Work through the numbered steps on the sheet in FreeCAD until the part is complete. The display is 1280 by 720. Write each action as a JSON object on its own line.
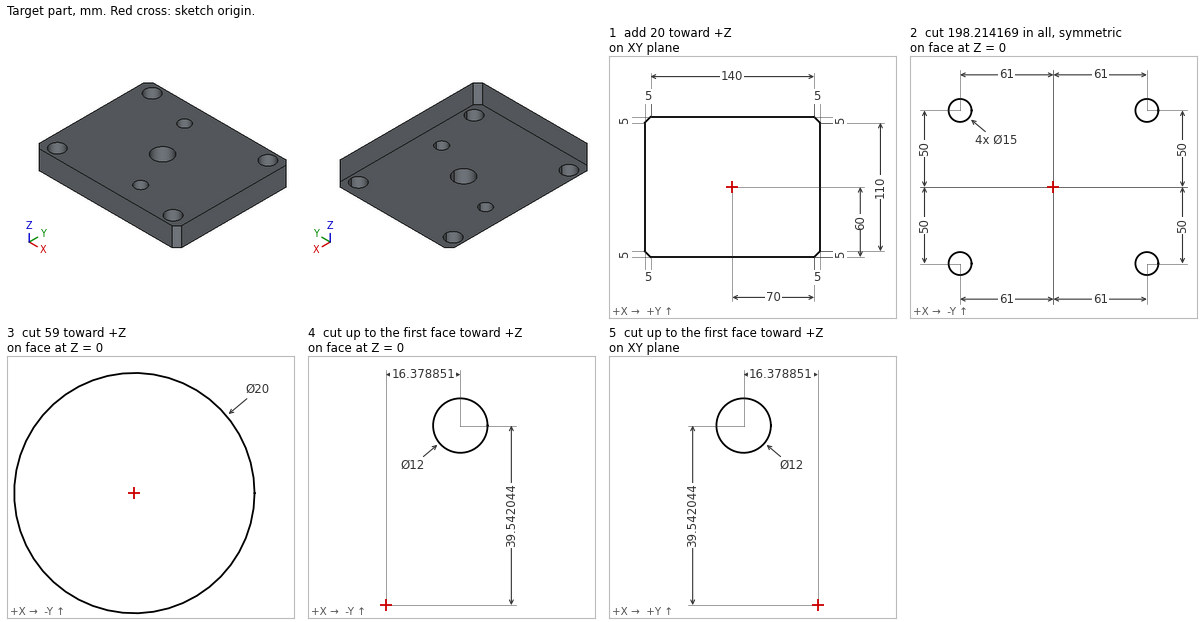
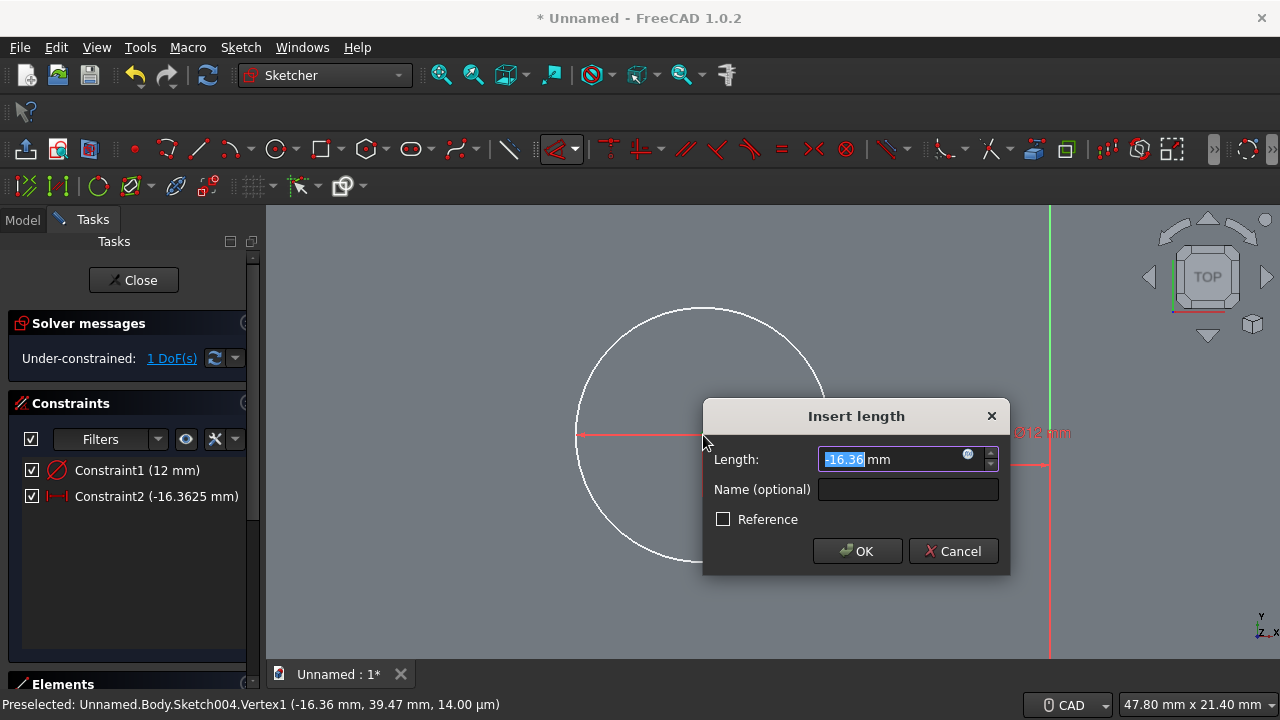
{"action": "type", "text": "-16.378851"}
{"action": "key", "text": "Return"}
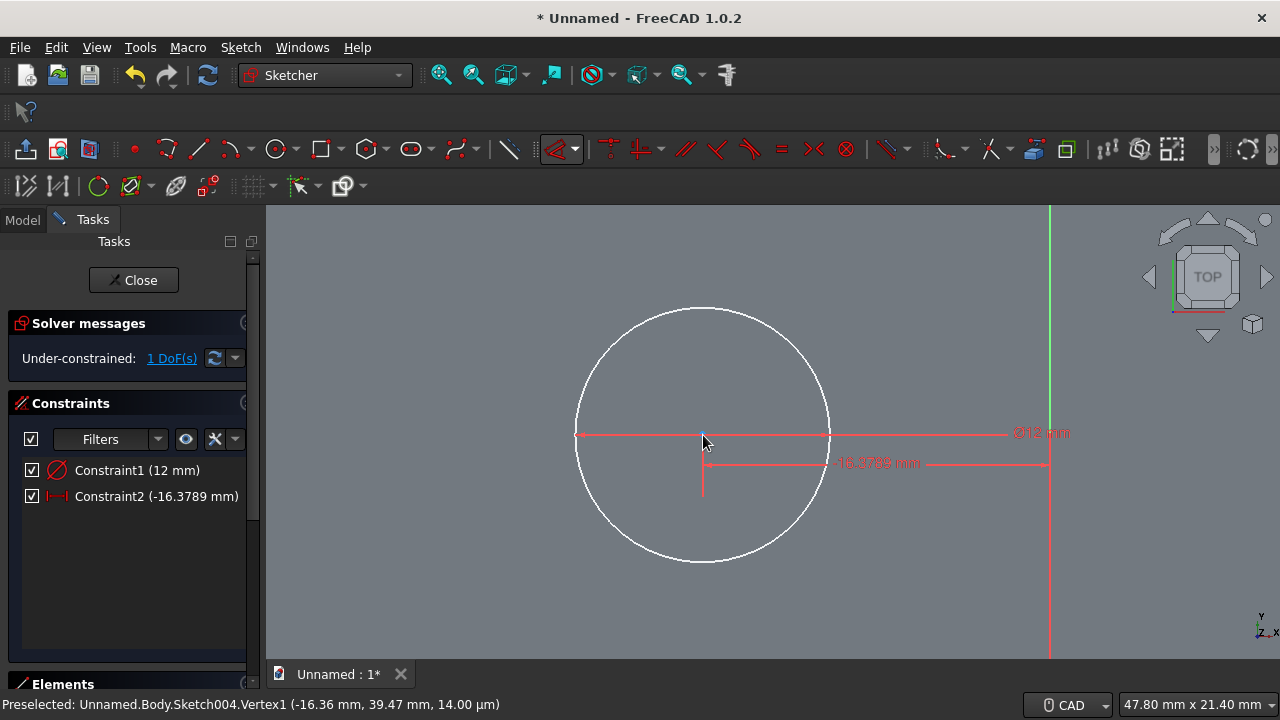
{"action": "left_click", "coordinate": [703, 435]}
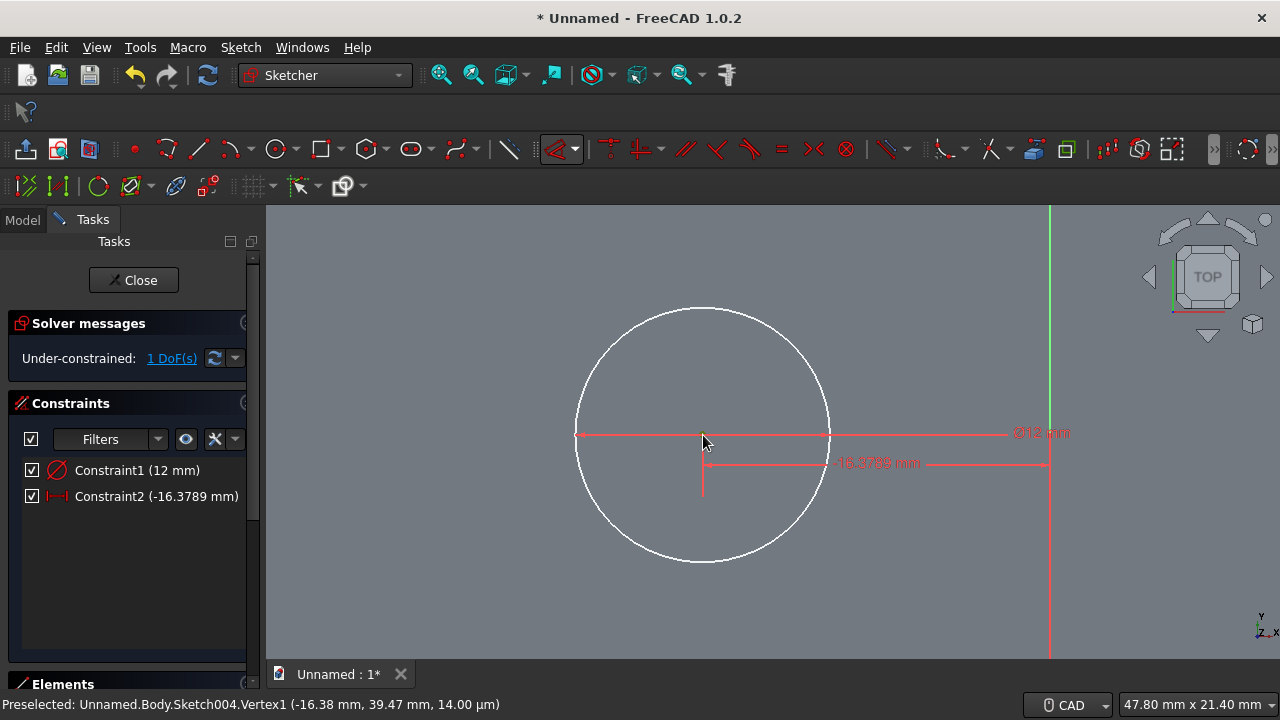
{"action": "left_click", "coordinate": [578, 150]}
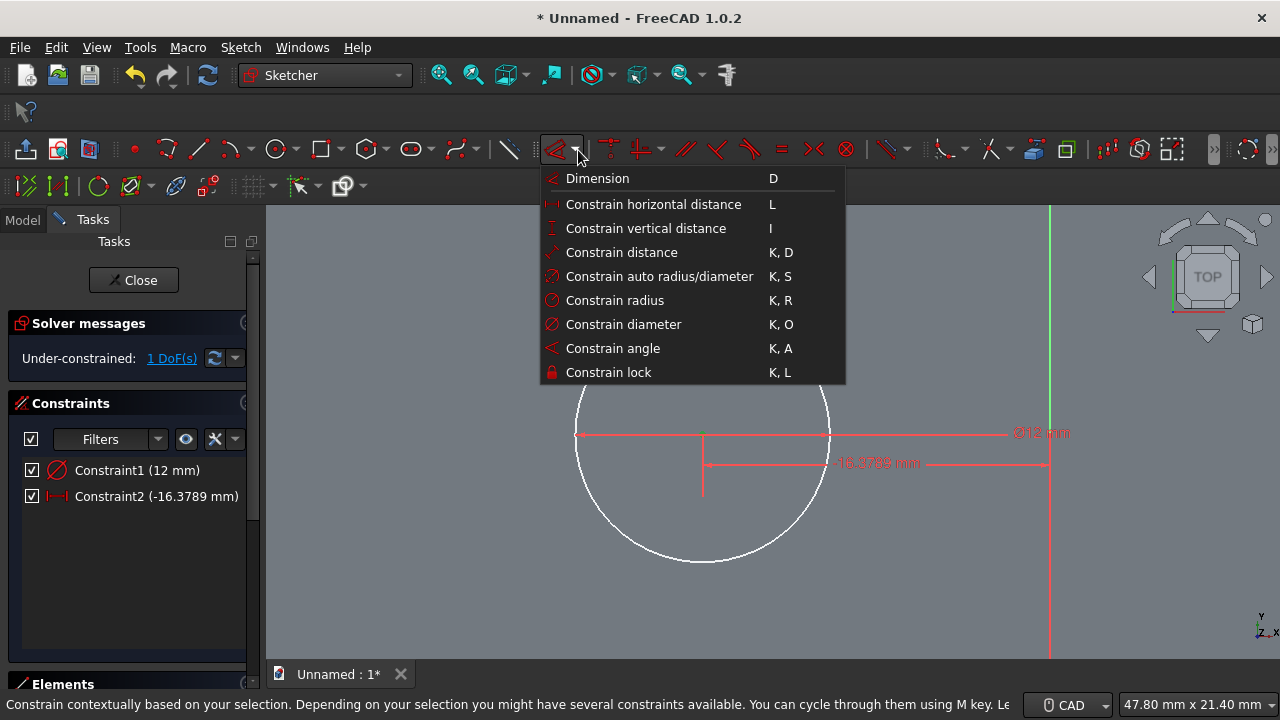
{"action": "left_click", "coordinate": [693, 228]}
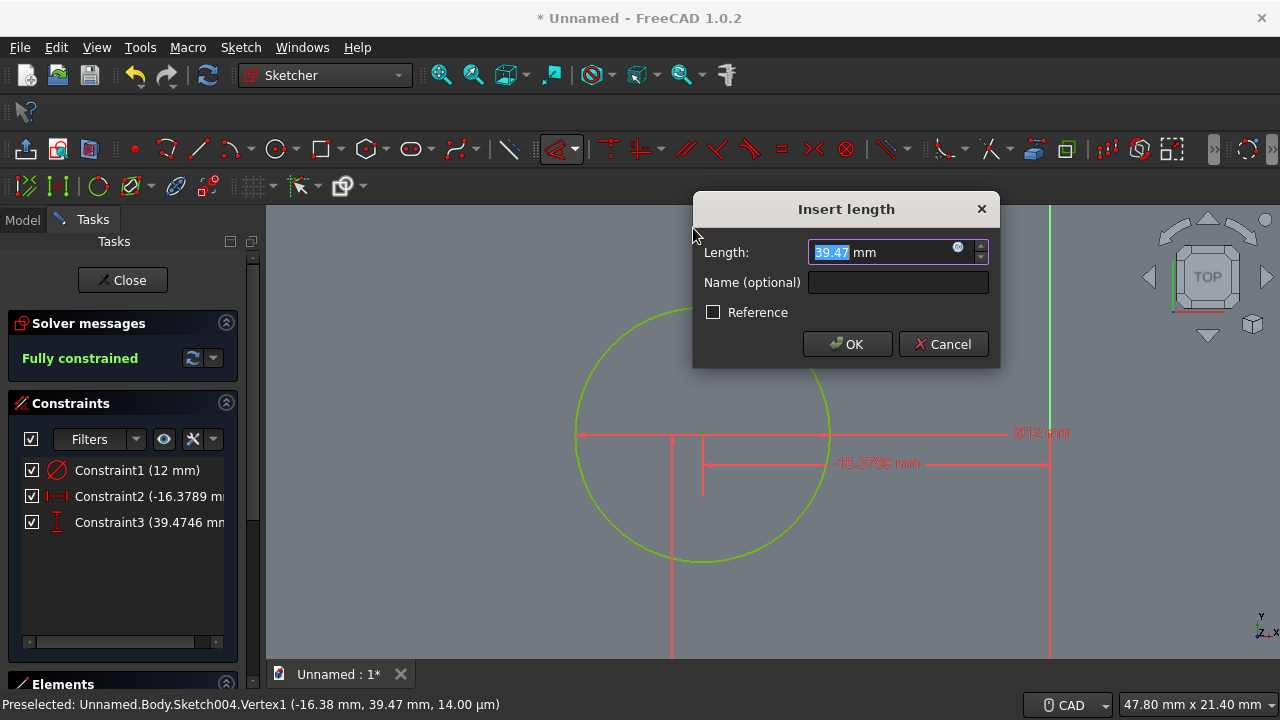
{"action": "type", "text": "39.542044"}
{"action": "key", "text": "Return"}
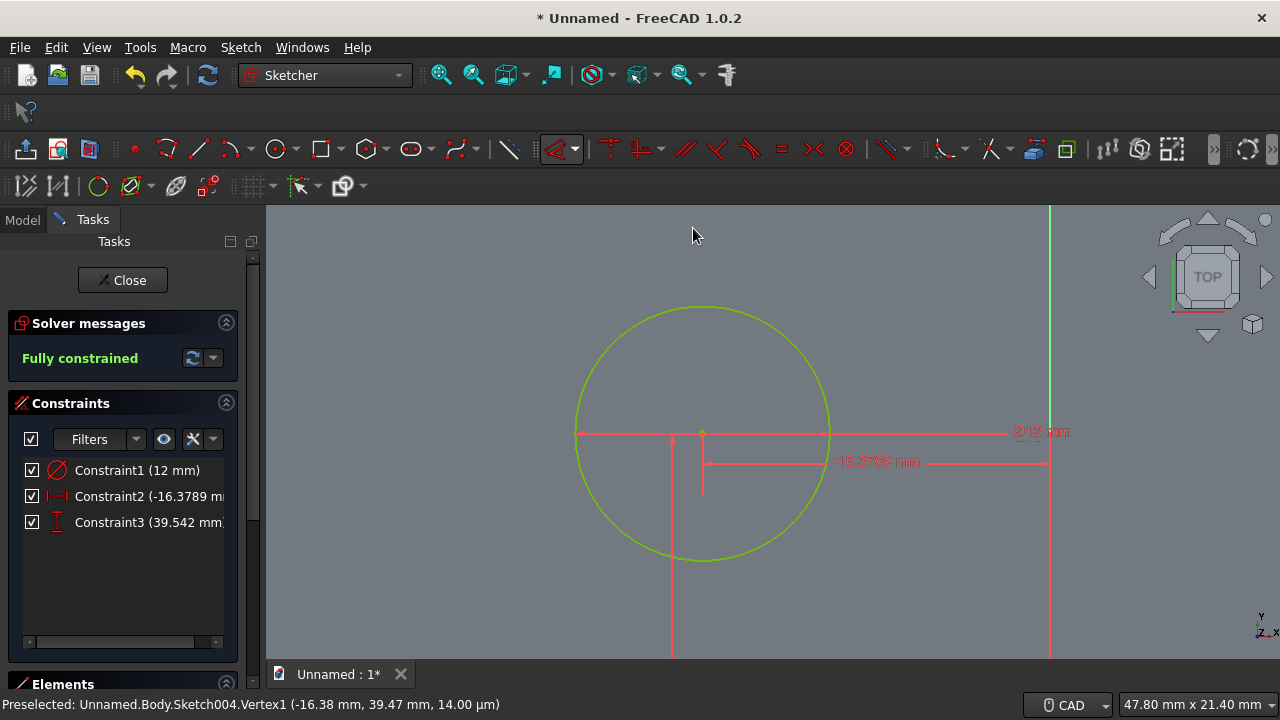
{"action": "left_click", "coordinate": [123, 280]}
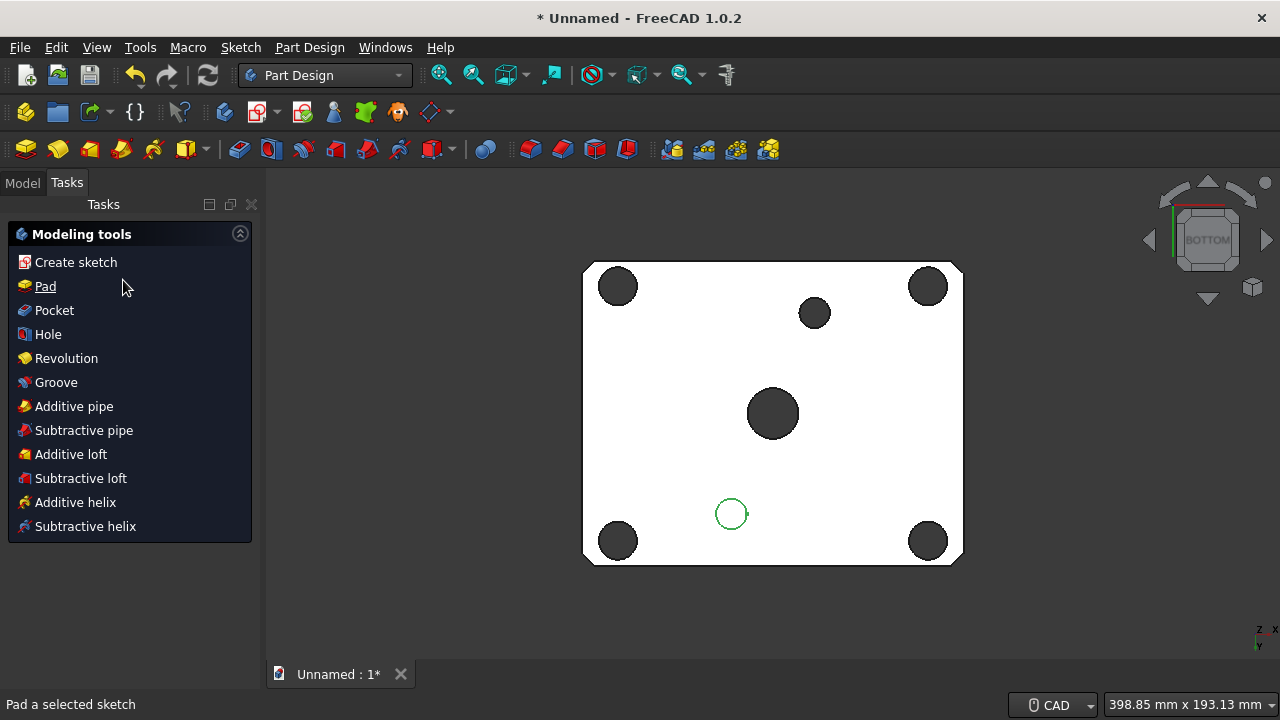
{"action": "left_click", "coordinate": [240, 150]}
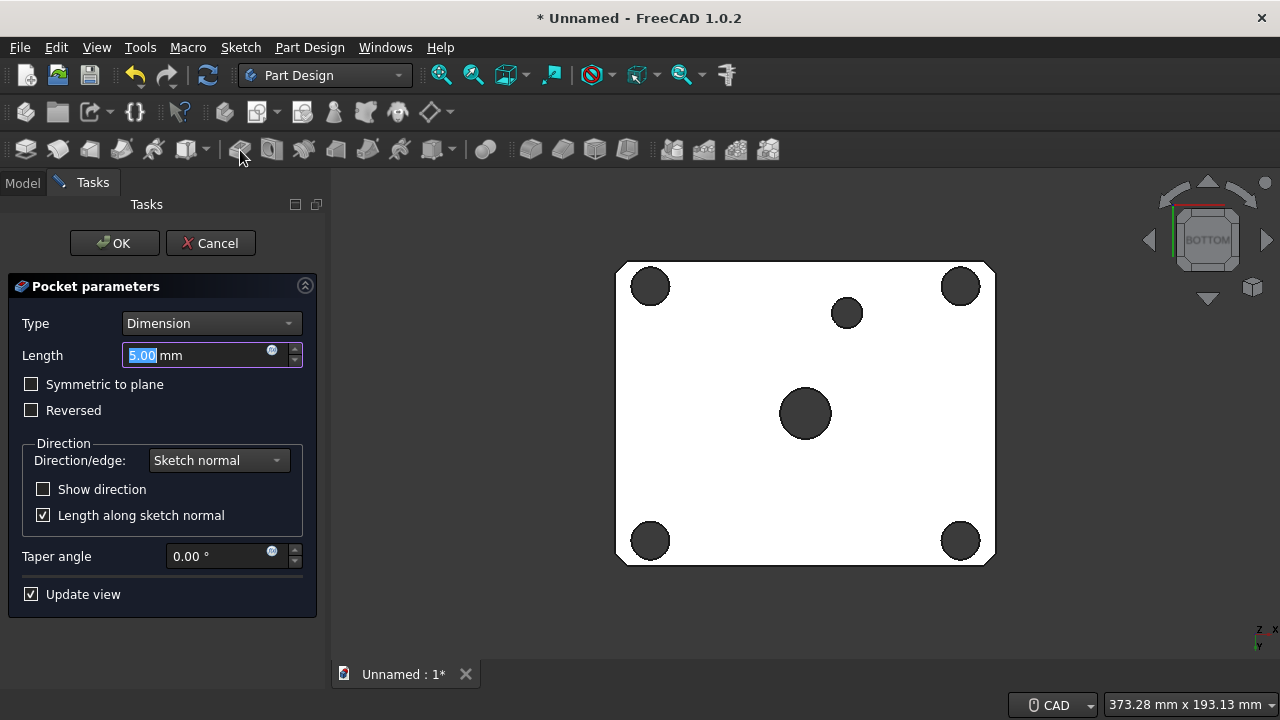
{"action": "left_click", "coordinate": [212, 324]}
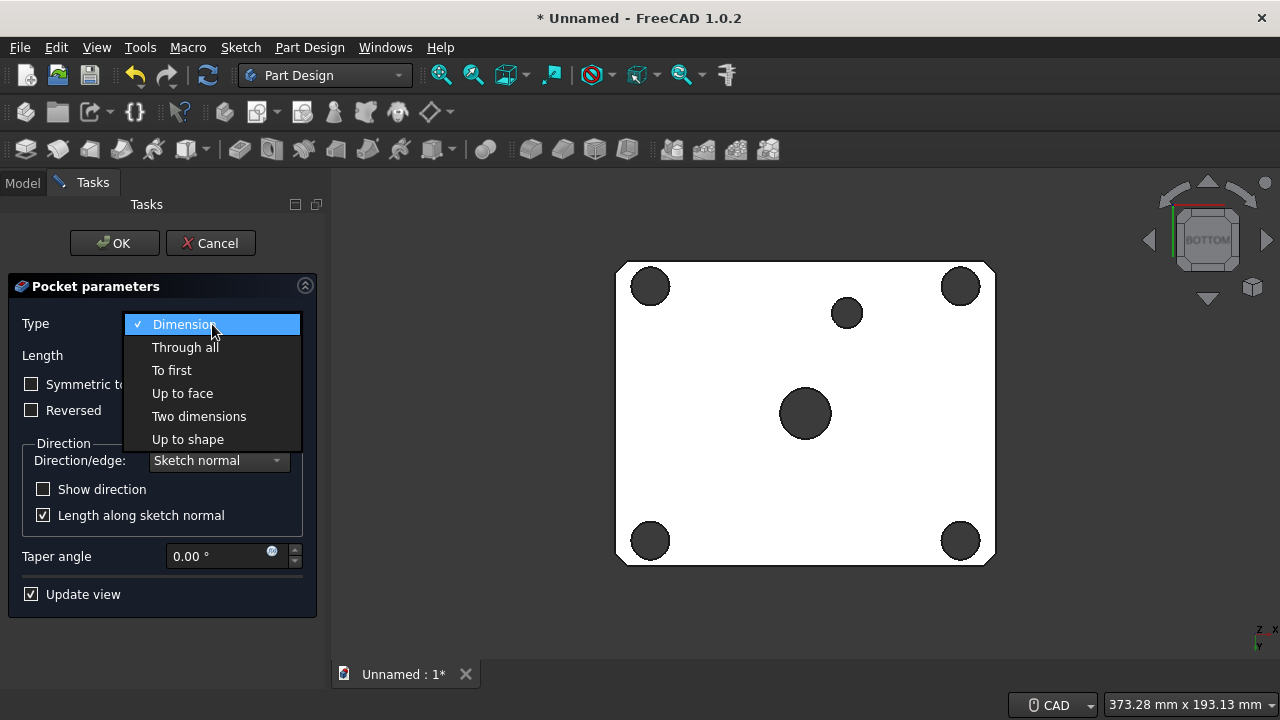
{"action": "left_click", "coordinate": [212, 370]}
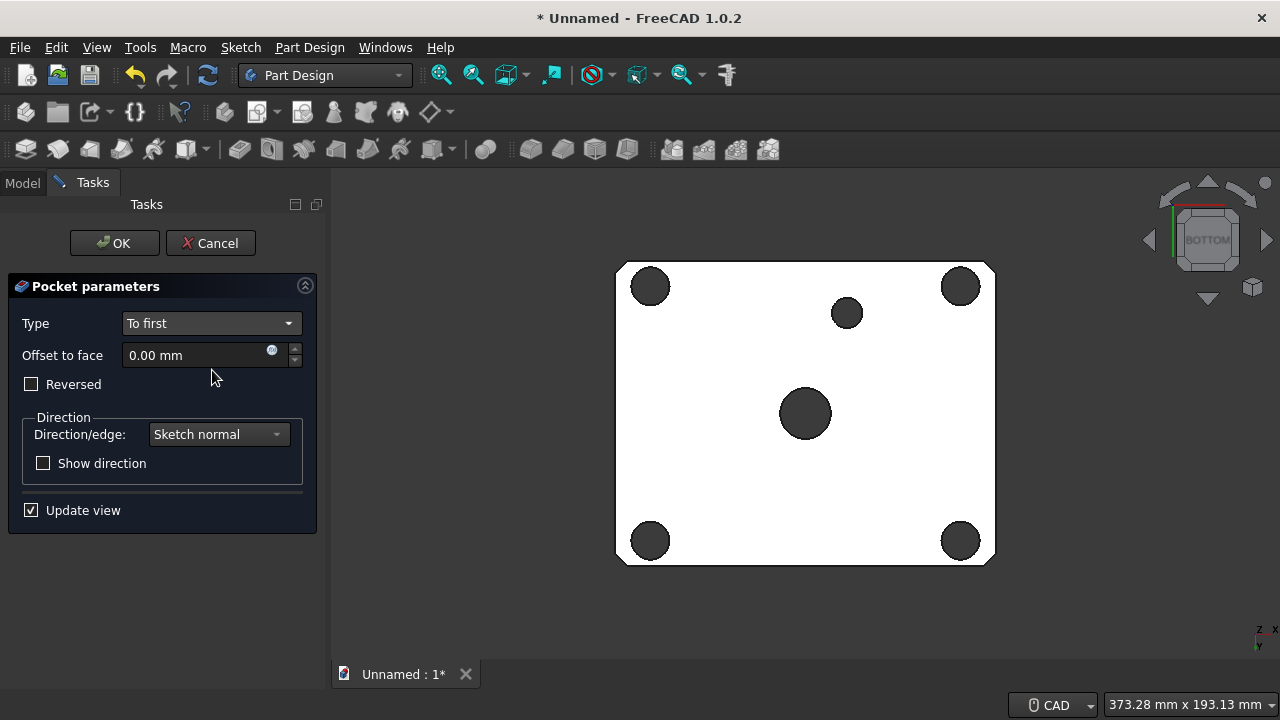
{"action": "left_click", "coordinate": [30, 384]}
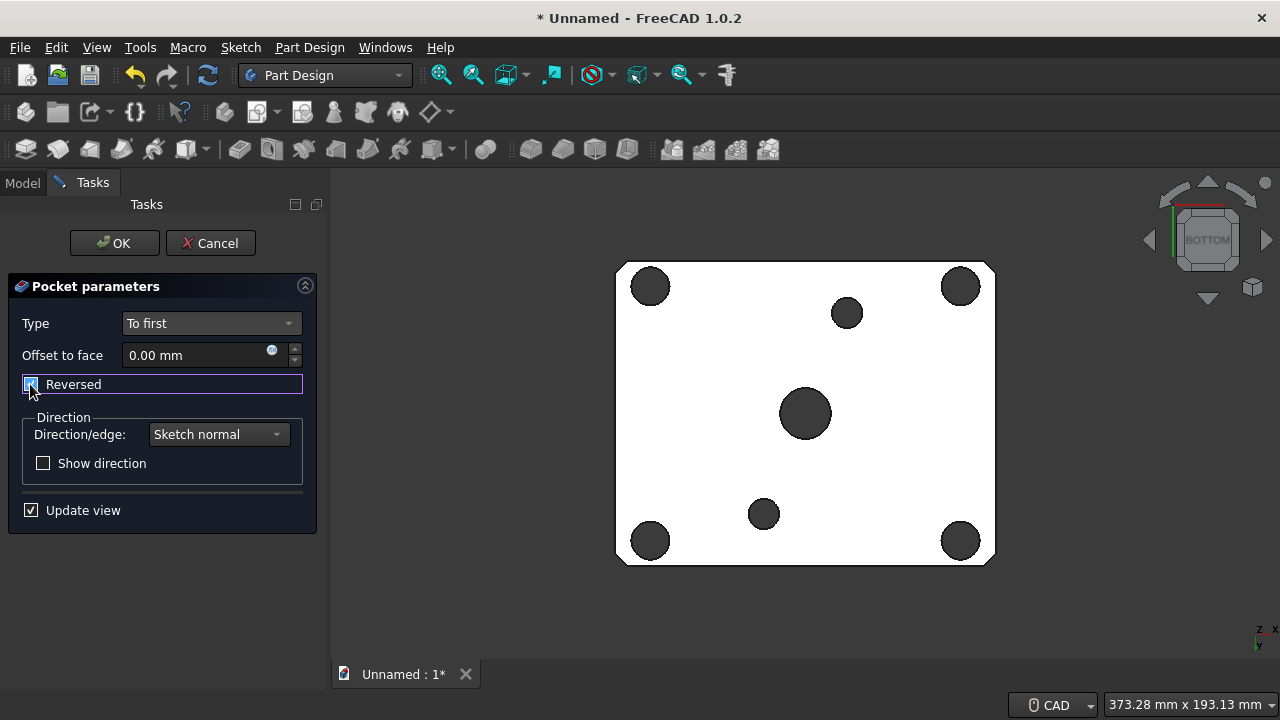
{"action": "left_click", "coordinate": [115, 243]}